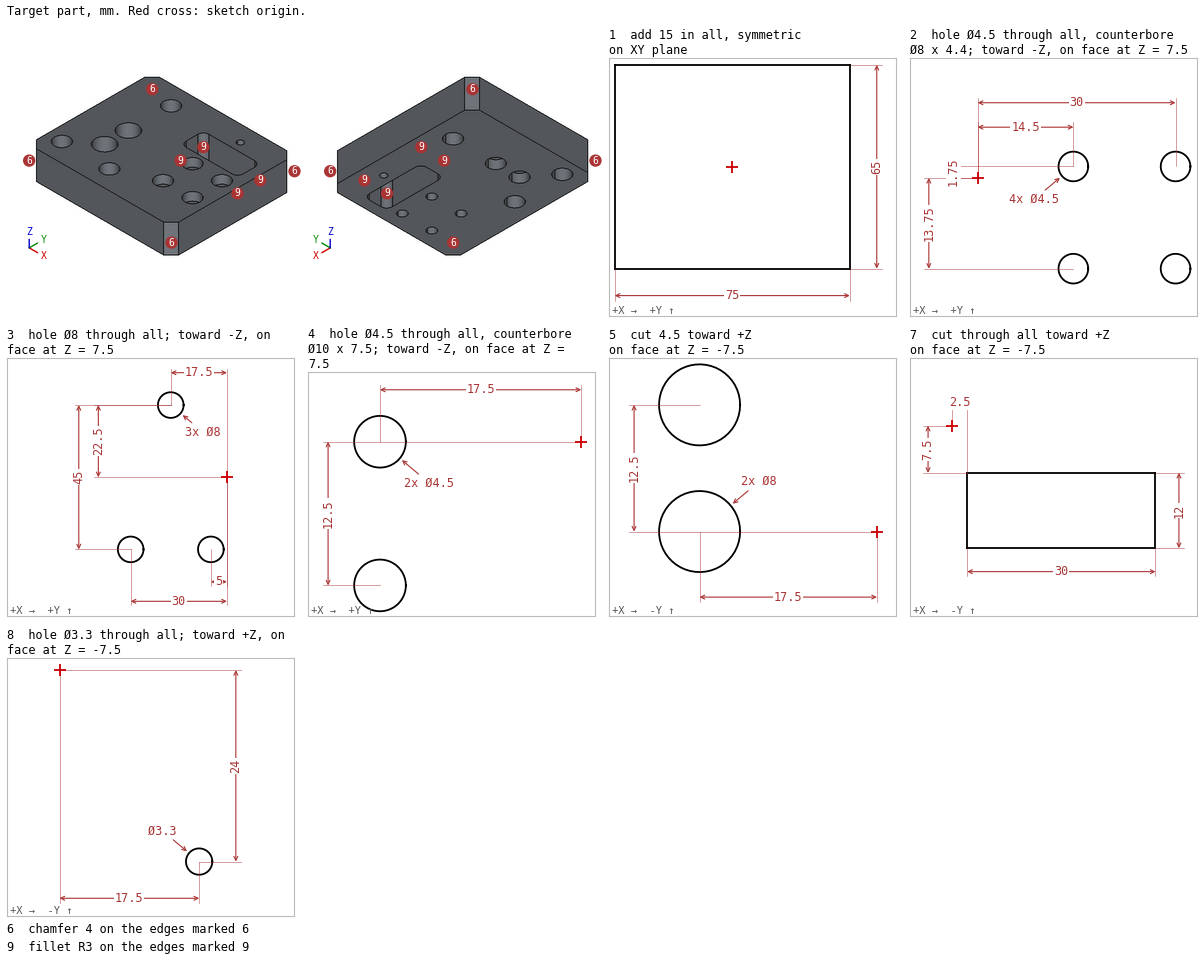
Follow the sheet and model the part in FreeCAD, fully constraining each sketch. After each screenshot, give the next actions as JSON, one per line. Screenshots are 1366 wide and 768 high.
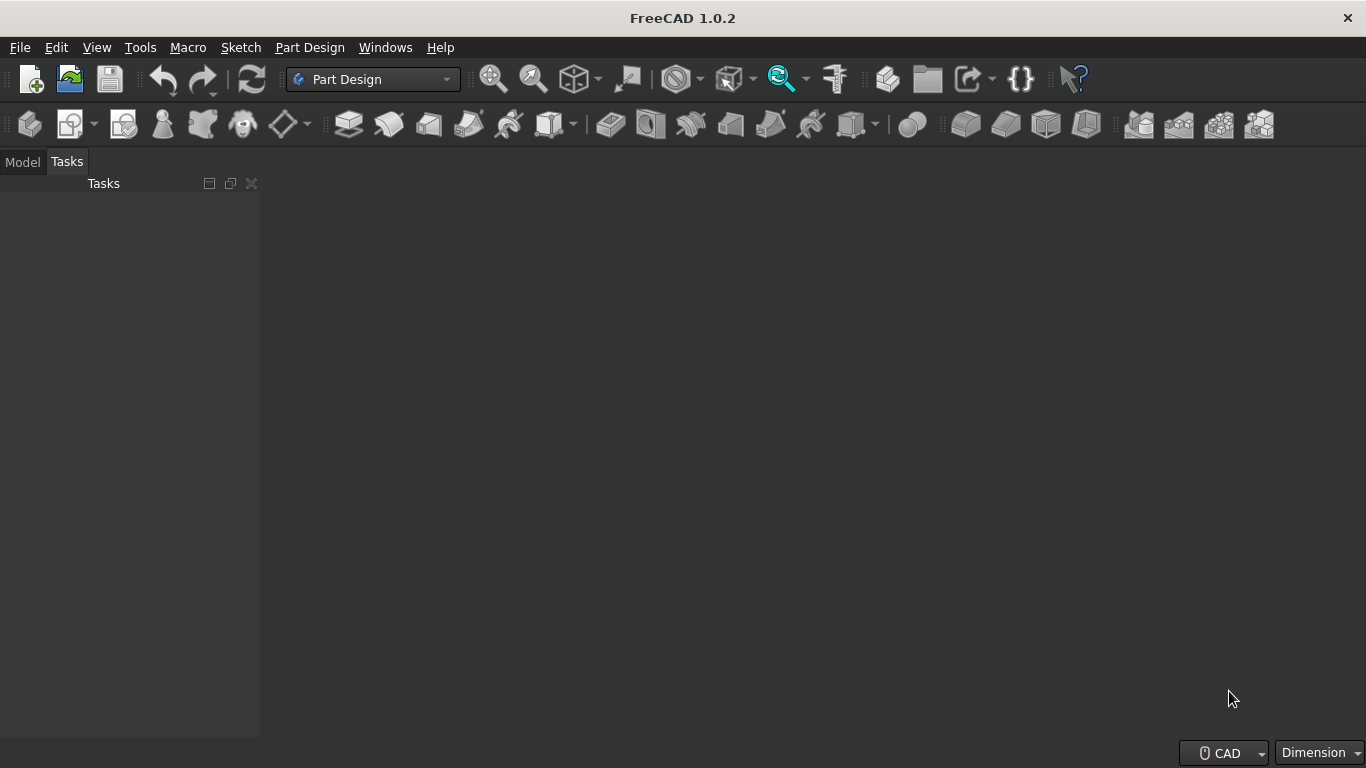
{"action": "left_click", "coordinate": [30, 80]}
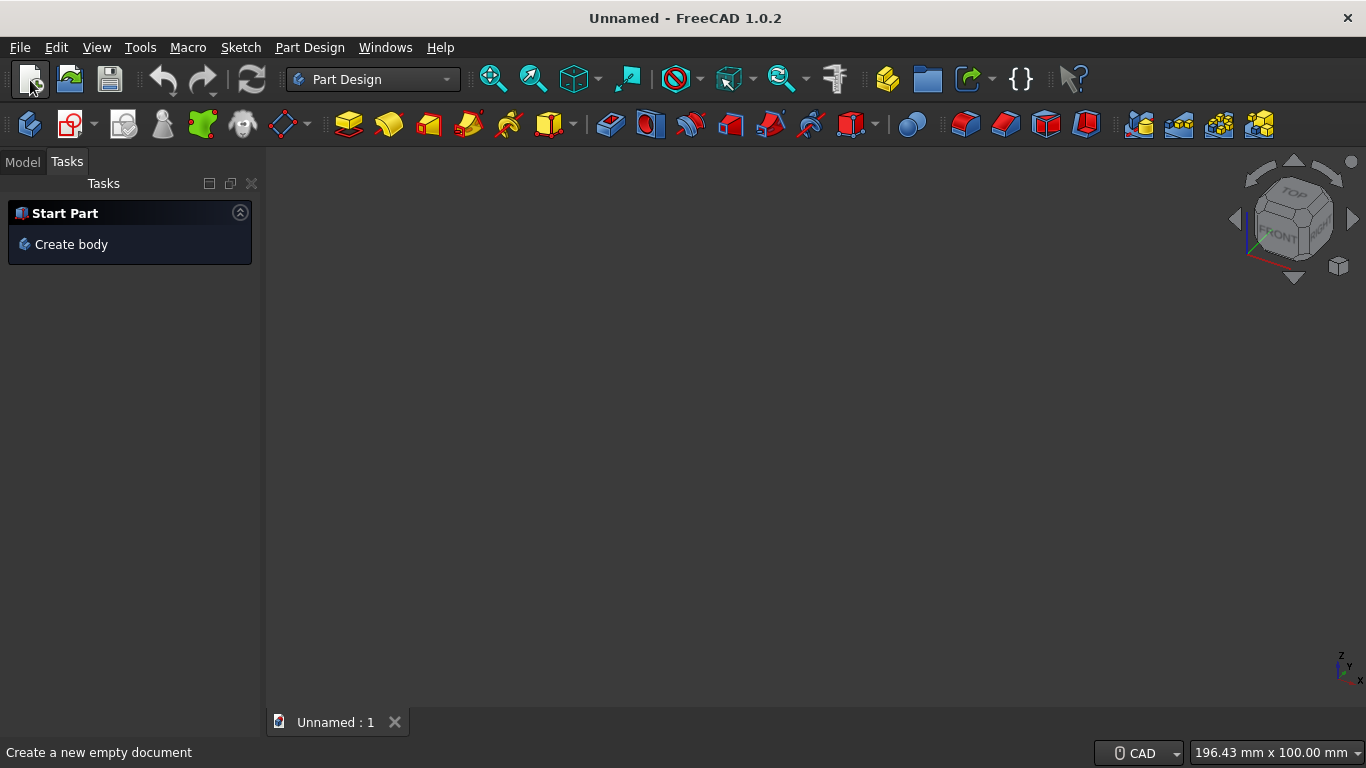
{"action": "left_click", "coordinate": [70, 124]}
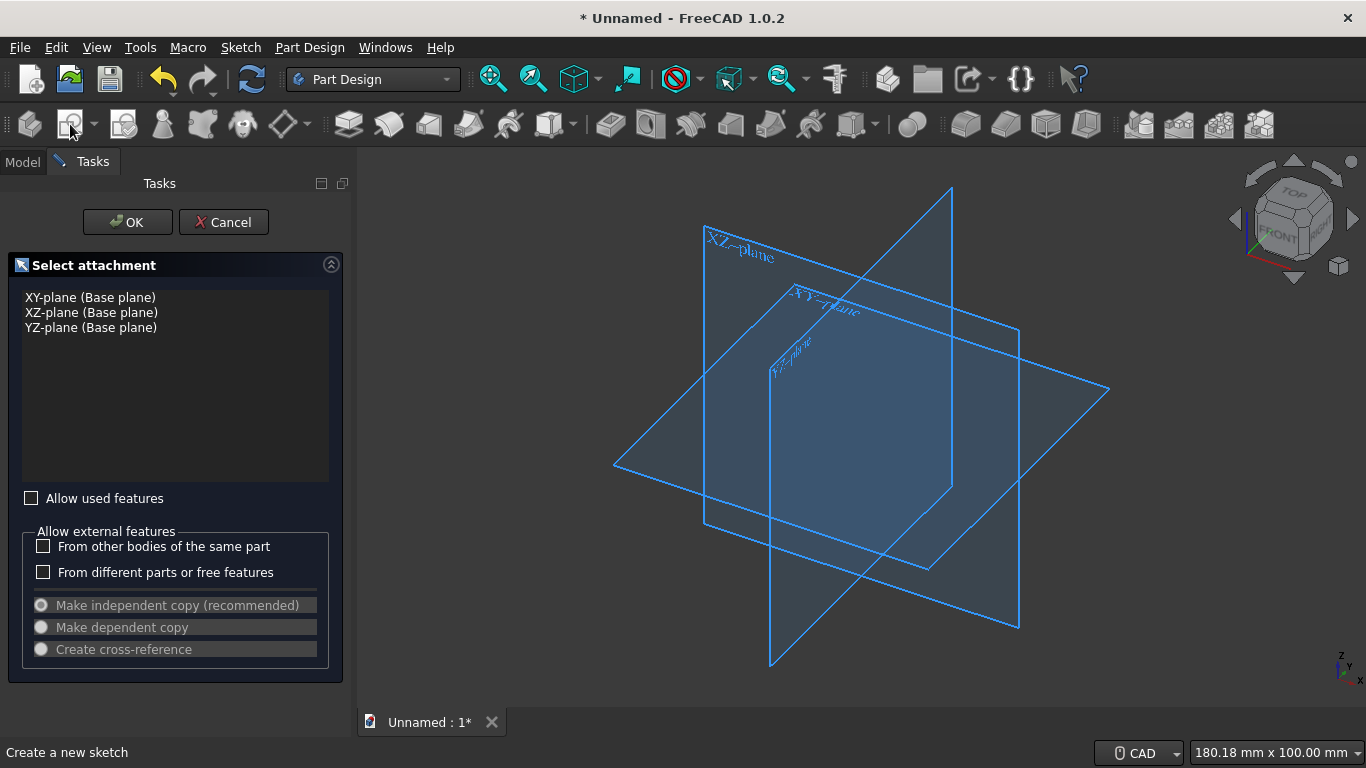
{"action": "left_click", "coordinate": [82, 298]}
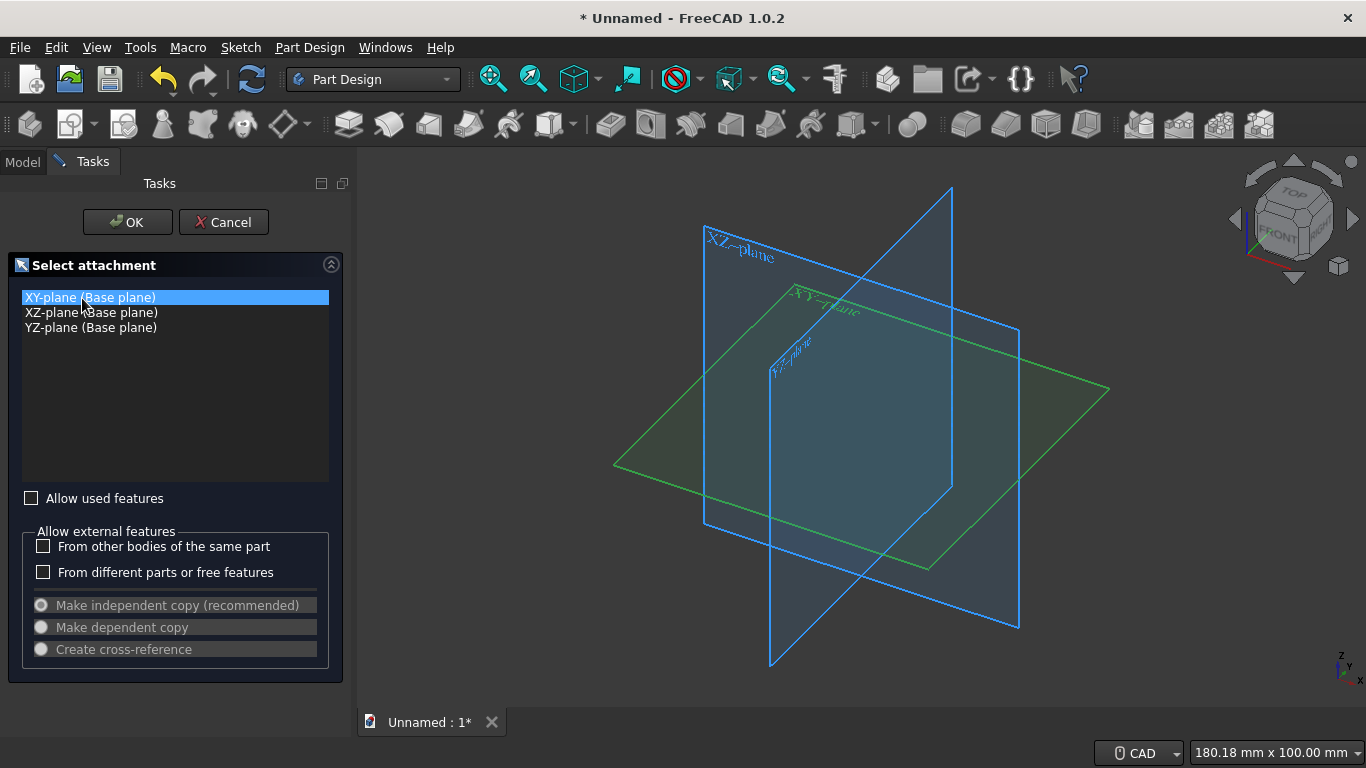
{"action": "left_click", "coordinate": [128, 222]}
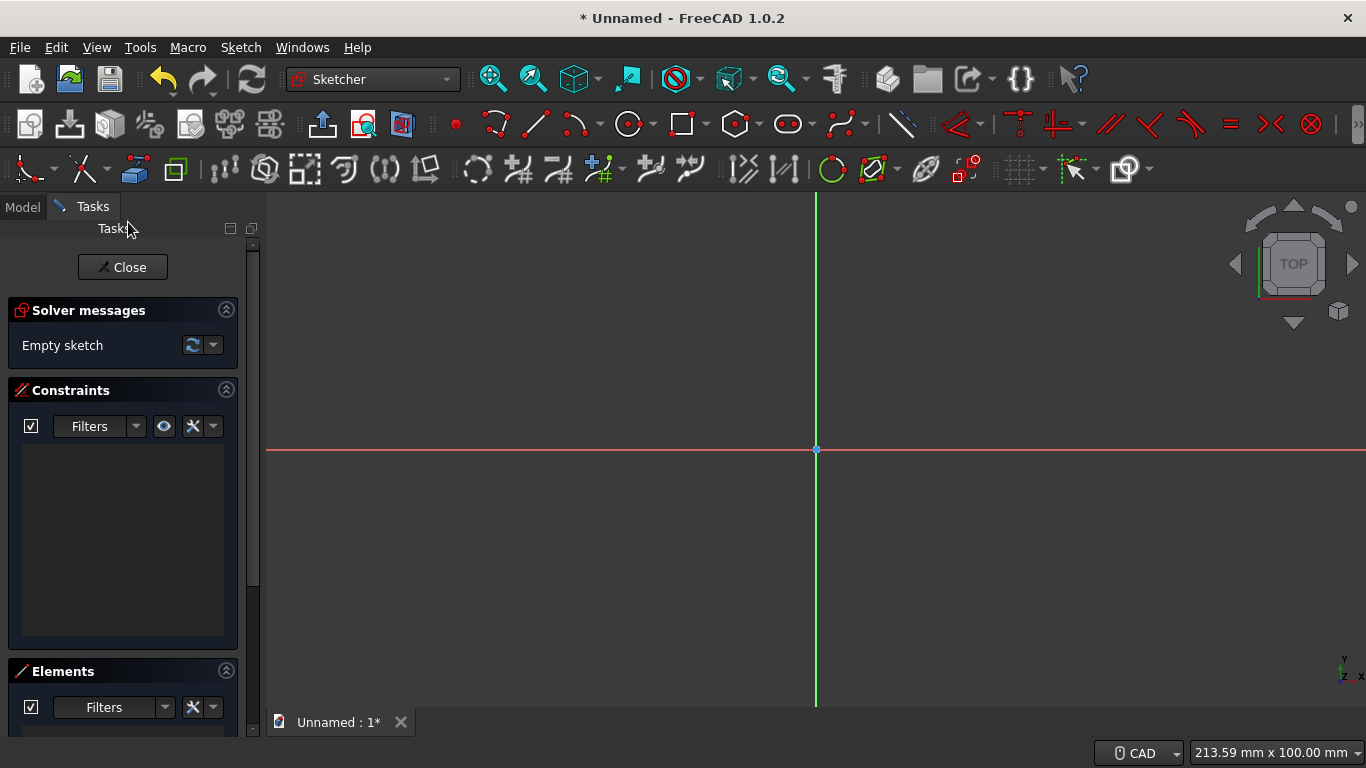
{"action": "left_click", "coordinate": [708, 124]}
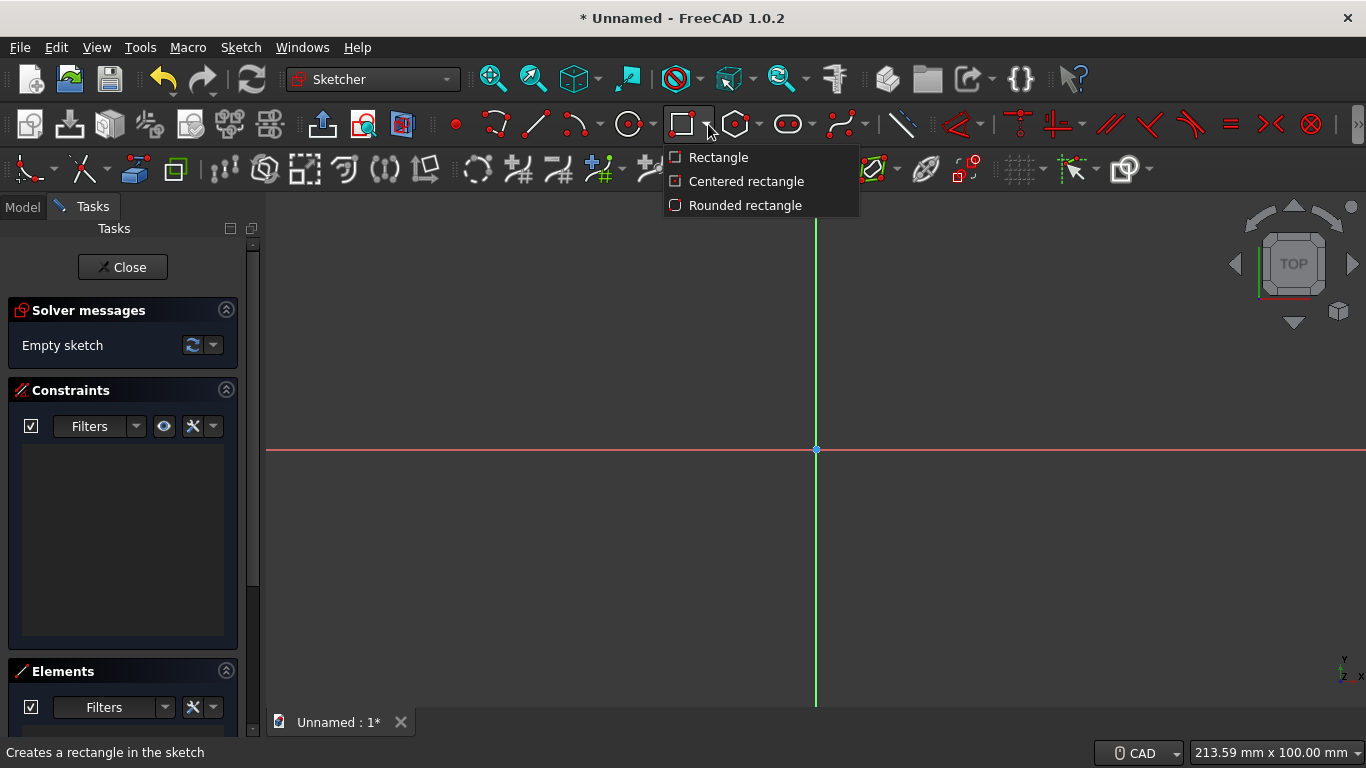
{"action": "left_click", "coordinate": [762, 181]}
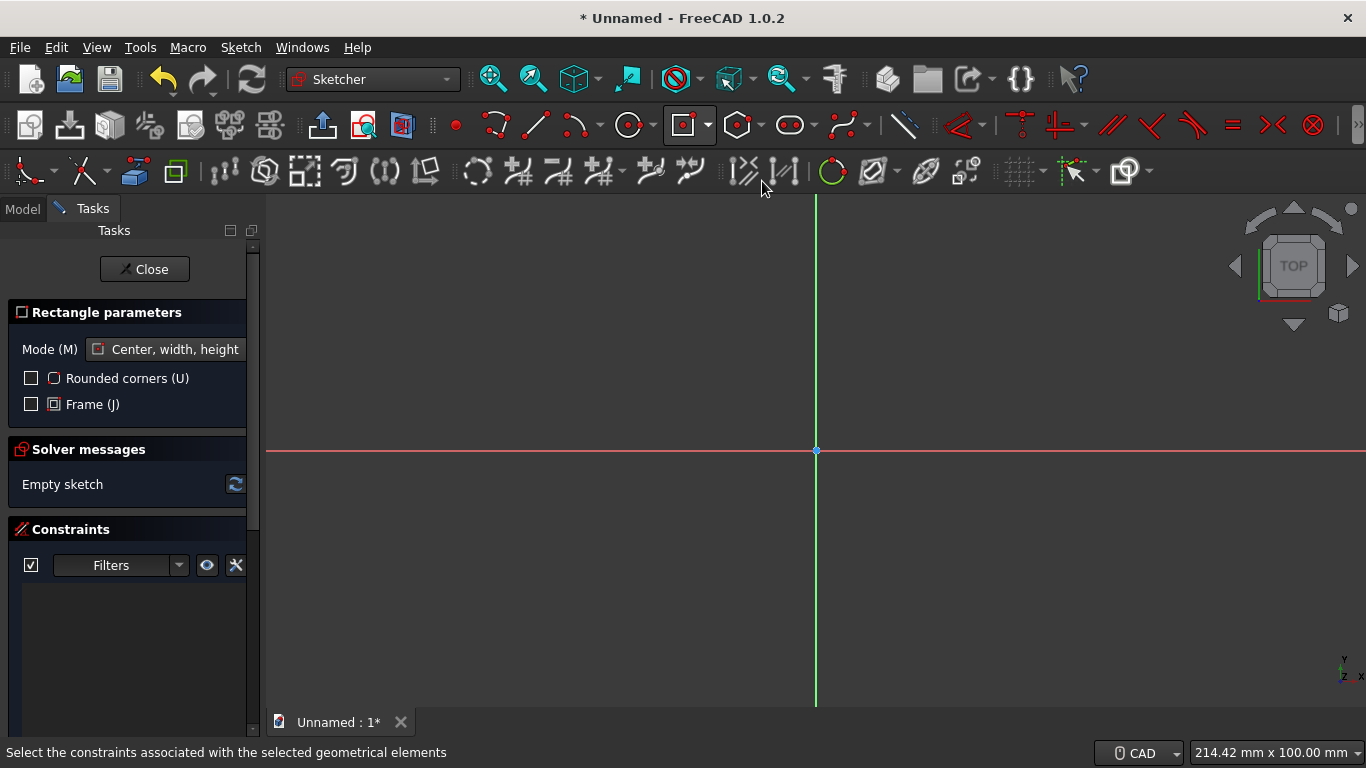
{"action": "left_click", "coordinate": [816, 450]}
{"action": "mouse_move", "coordinate": [1008, 284]}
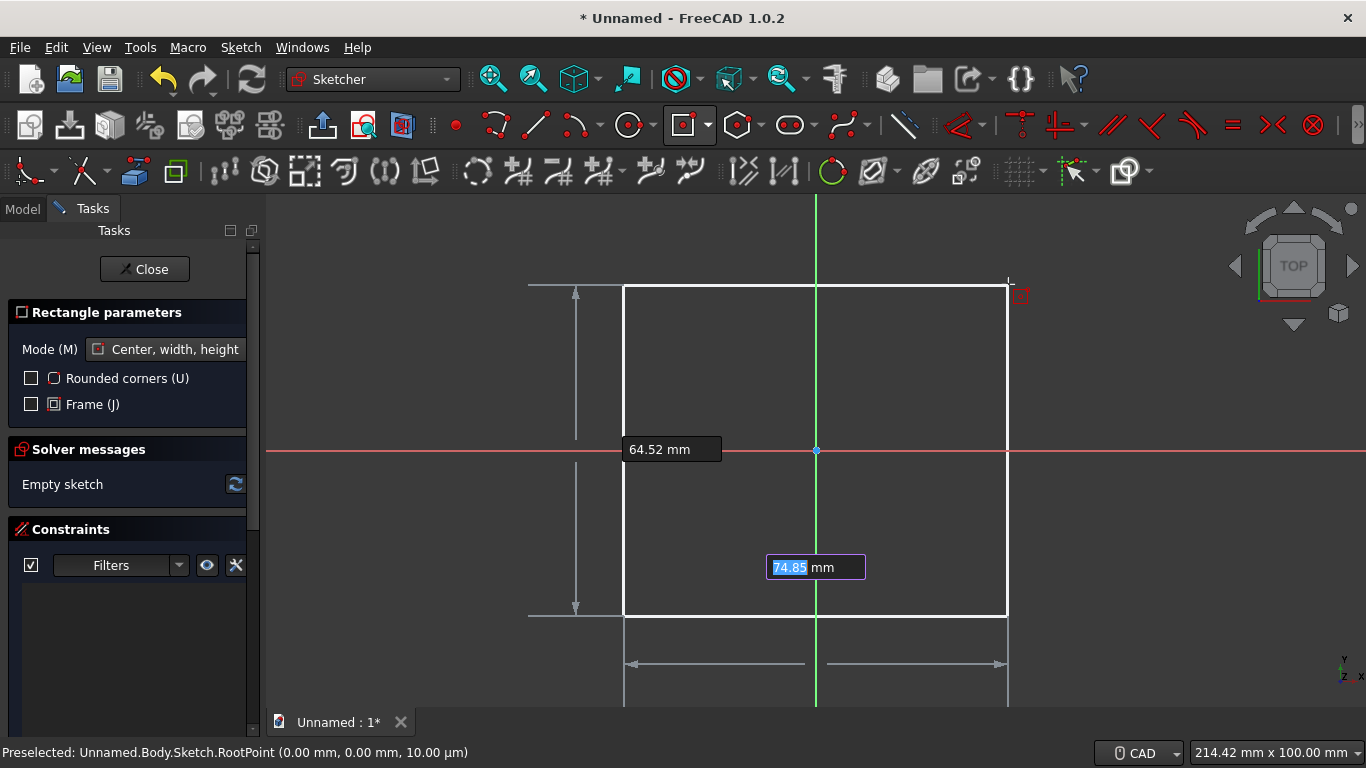
{"action": "type", "text": "75"}
{"action": "key", "text": "Tab"}
{"action": "type", "text": "65"}
{"action": "key", "text": "Return"}
{"action": "key", "text": "Escape"}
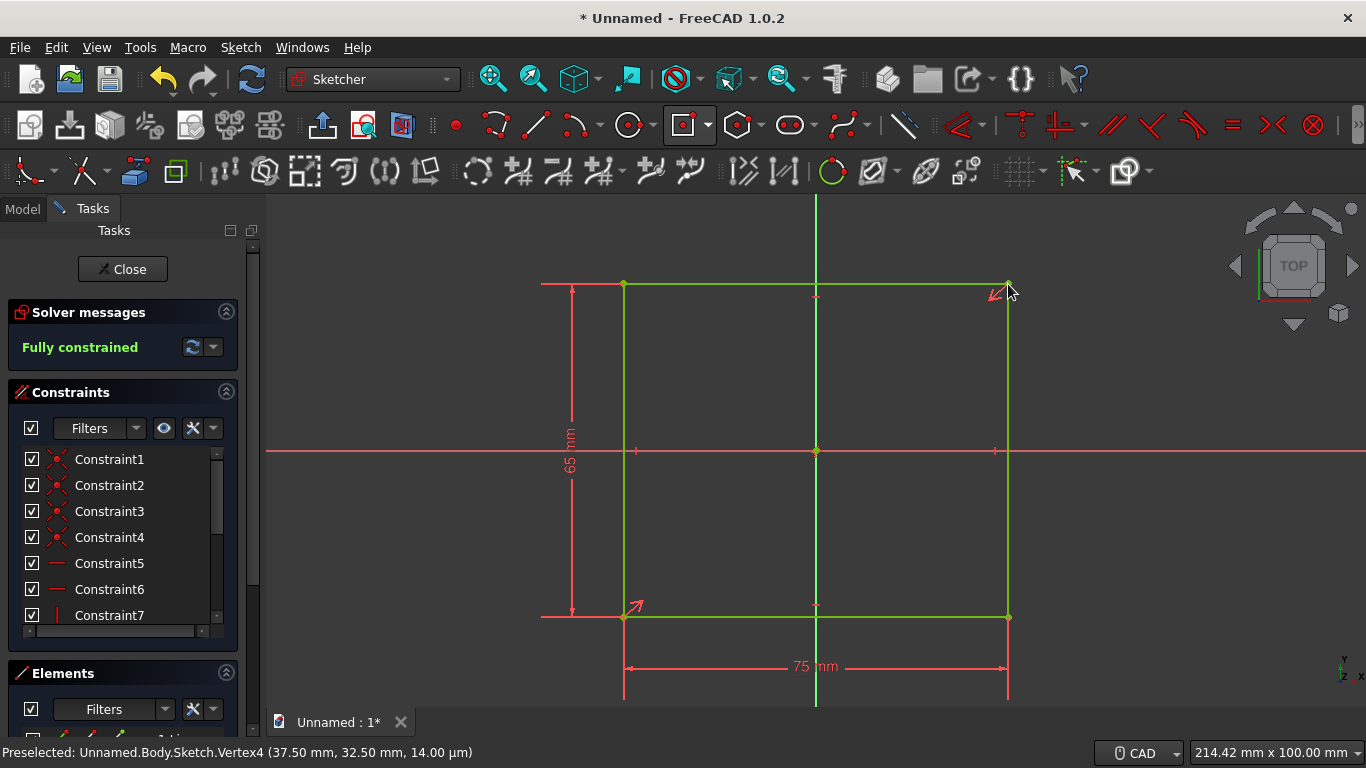
{"action": "left_click", "coordinate": [123, 269]}